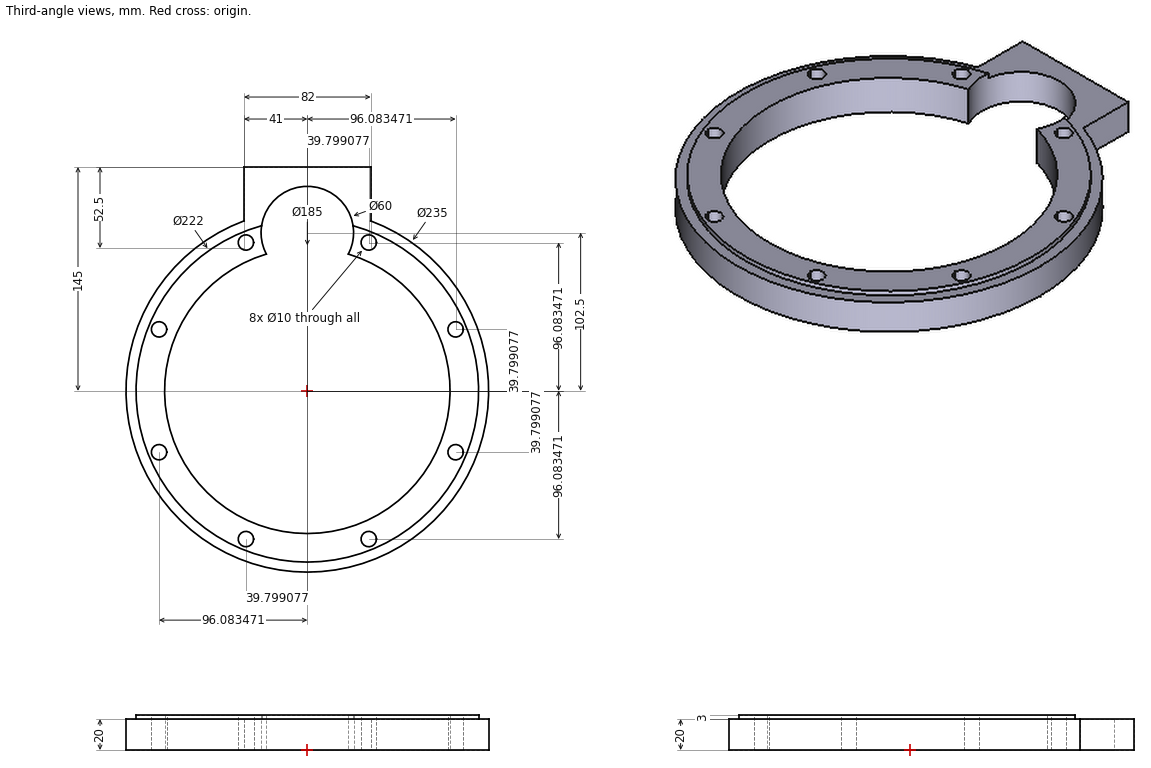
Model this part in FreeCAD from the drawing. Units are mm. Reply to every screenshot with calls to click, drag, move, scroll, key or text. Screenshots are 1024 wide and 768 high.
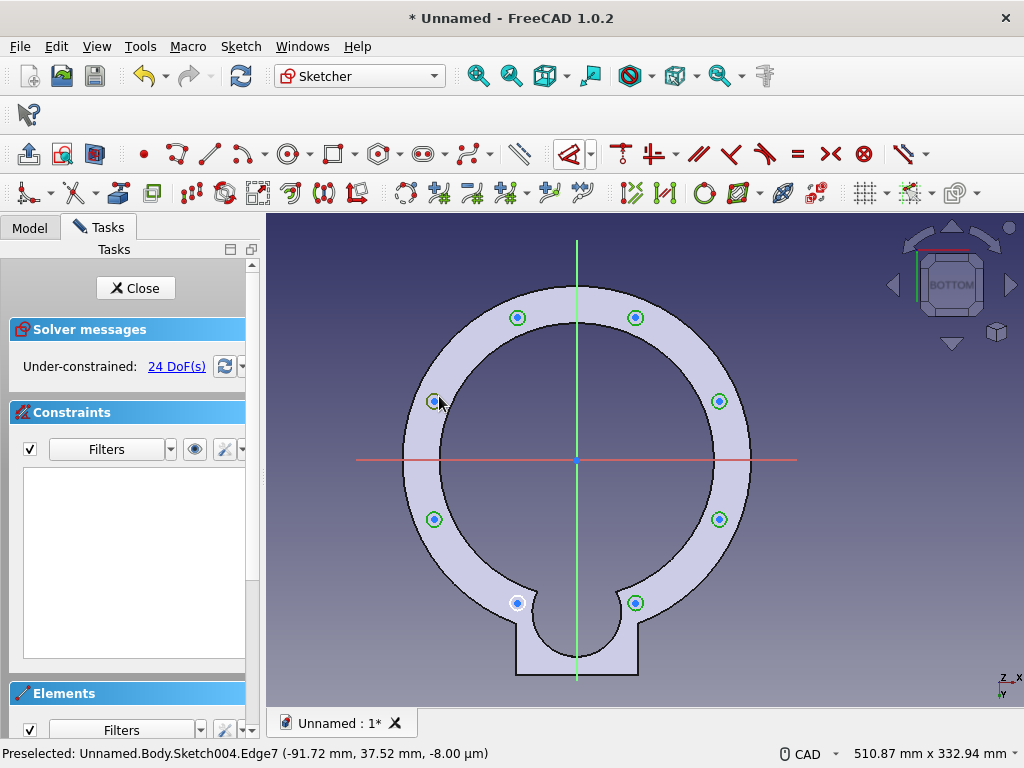
scroll(523, 598, up, 4)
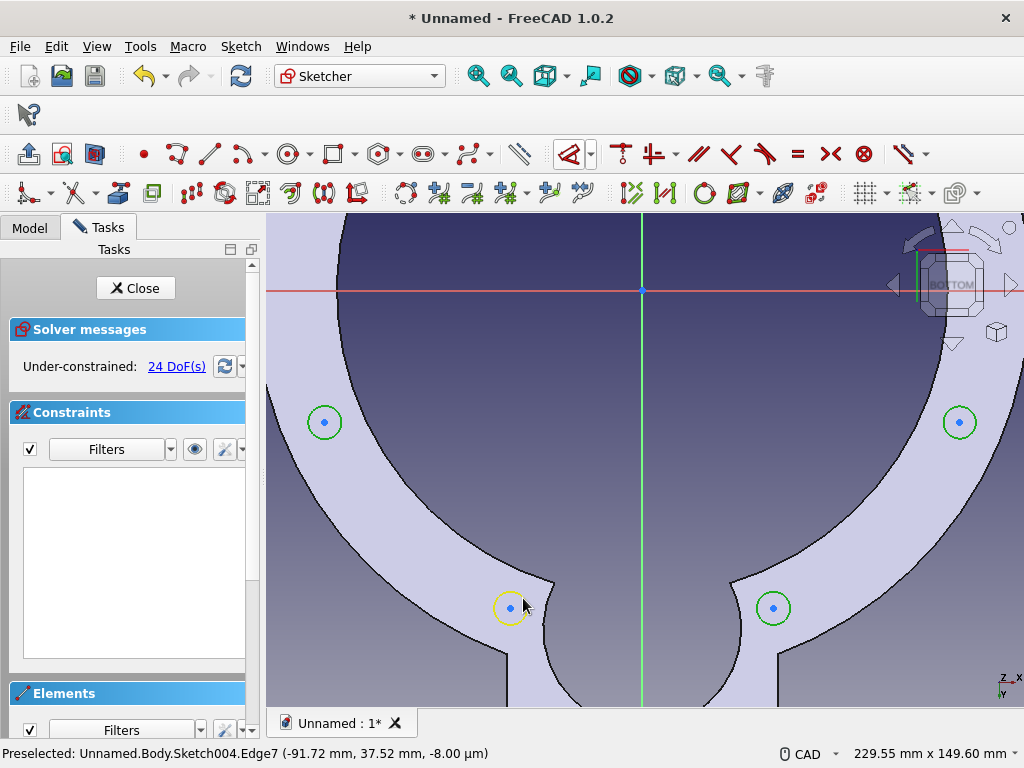
click(522, 597)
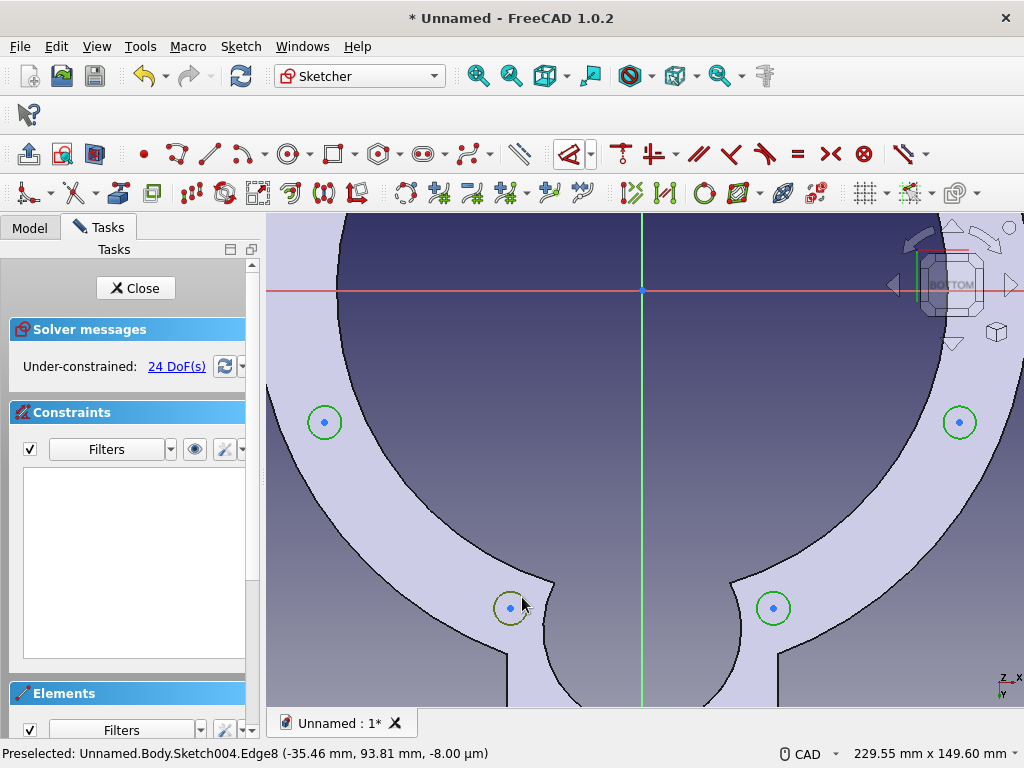
click(798, 154)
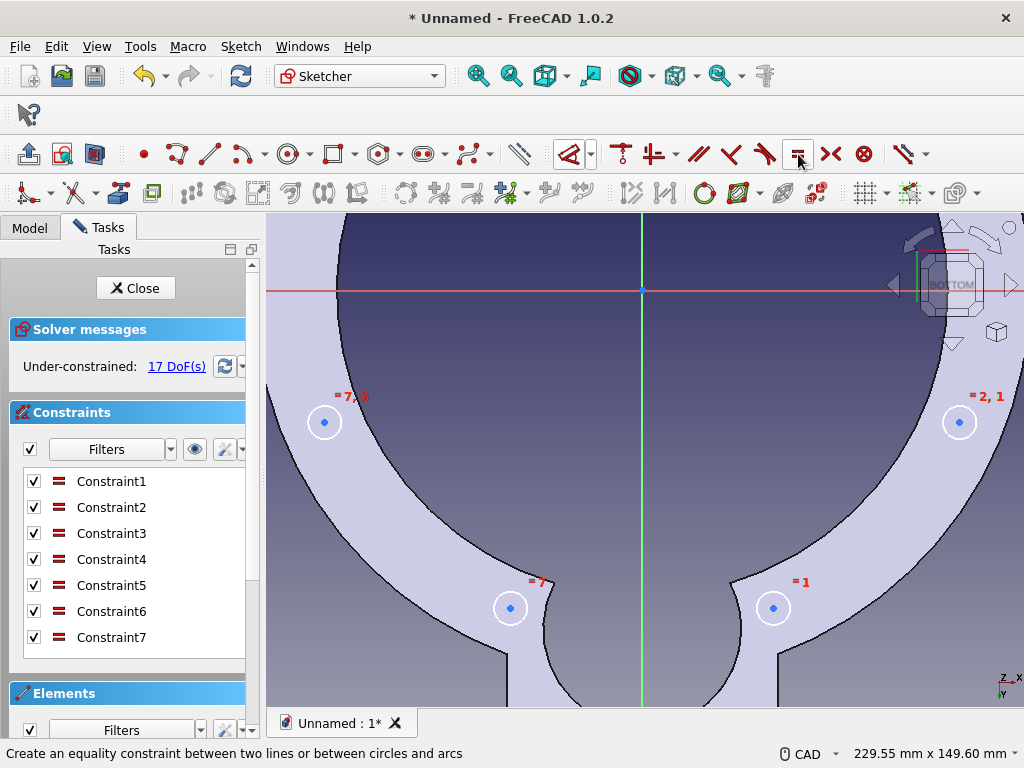
scroll(523, 598, down, 4)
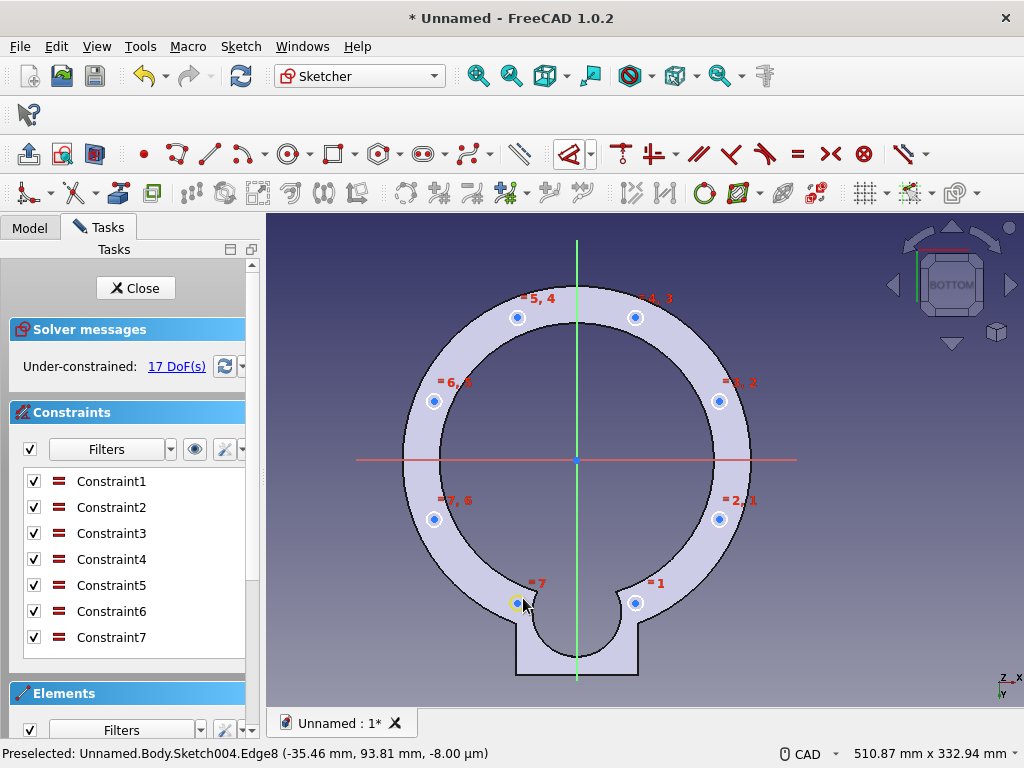
click(719, 520)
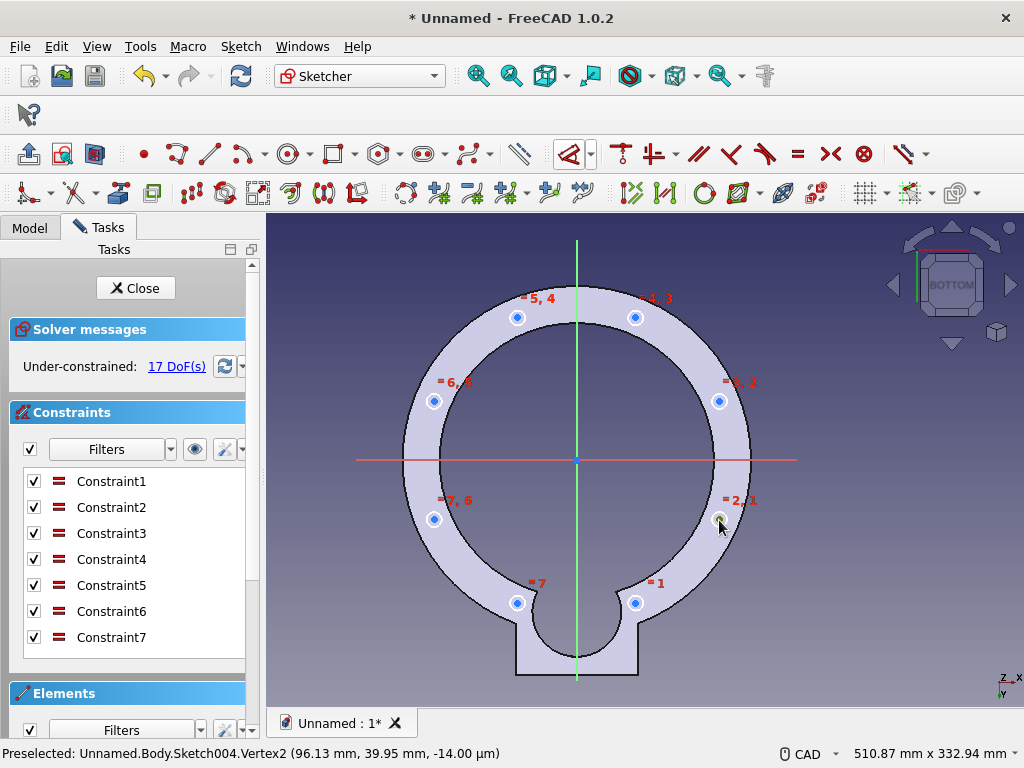
click(719, 401)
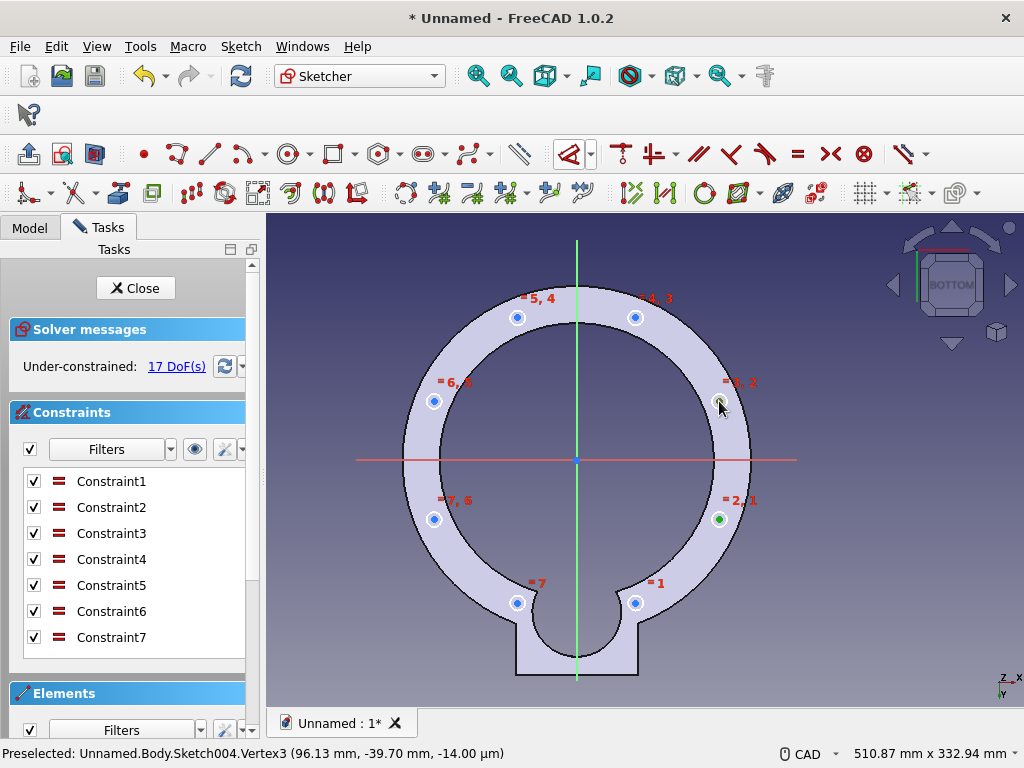
click(676, 154)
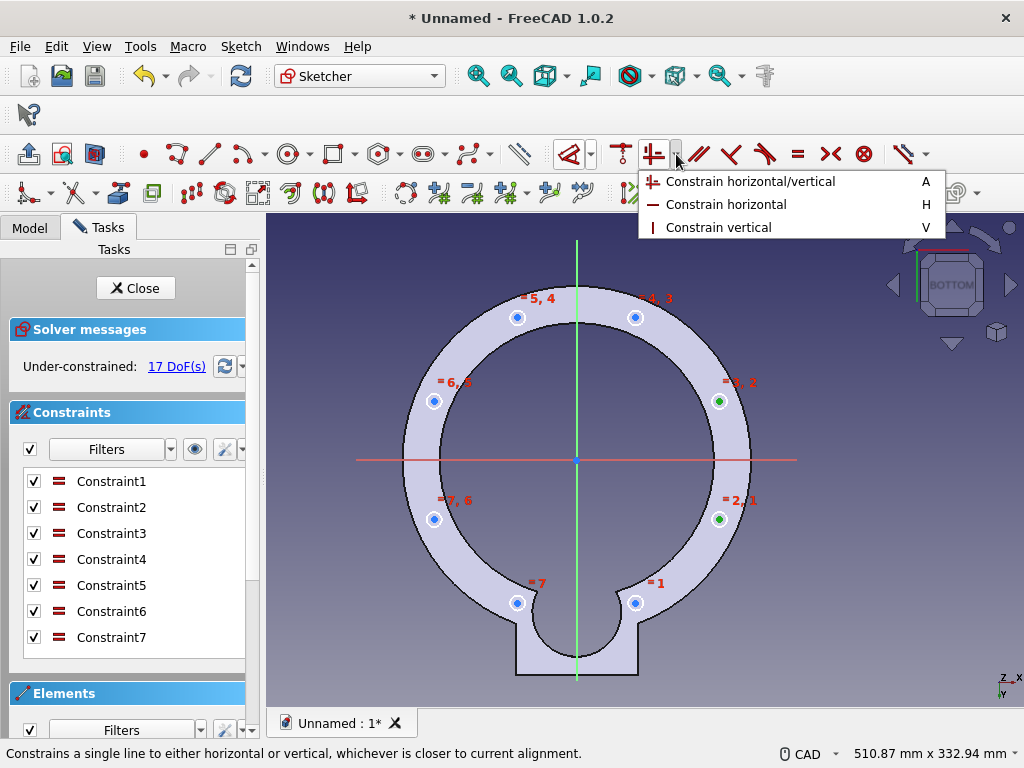
click(792, 228)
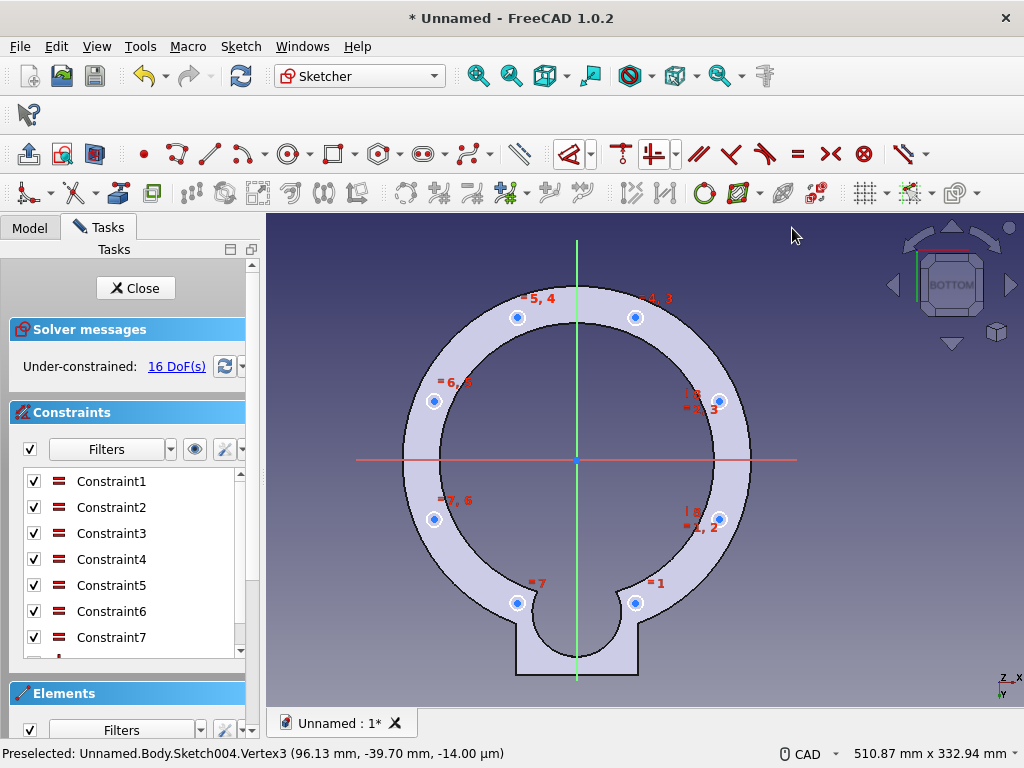
click(636, 603)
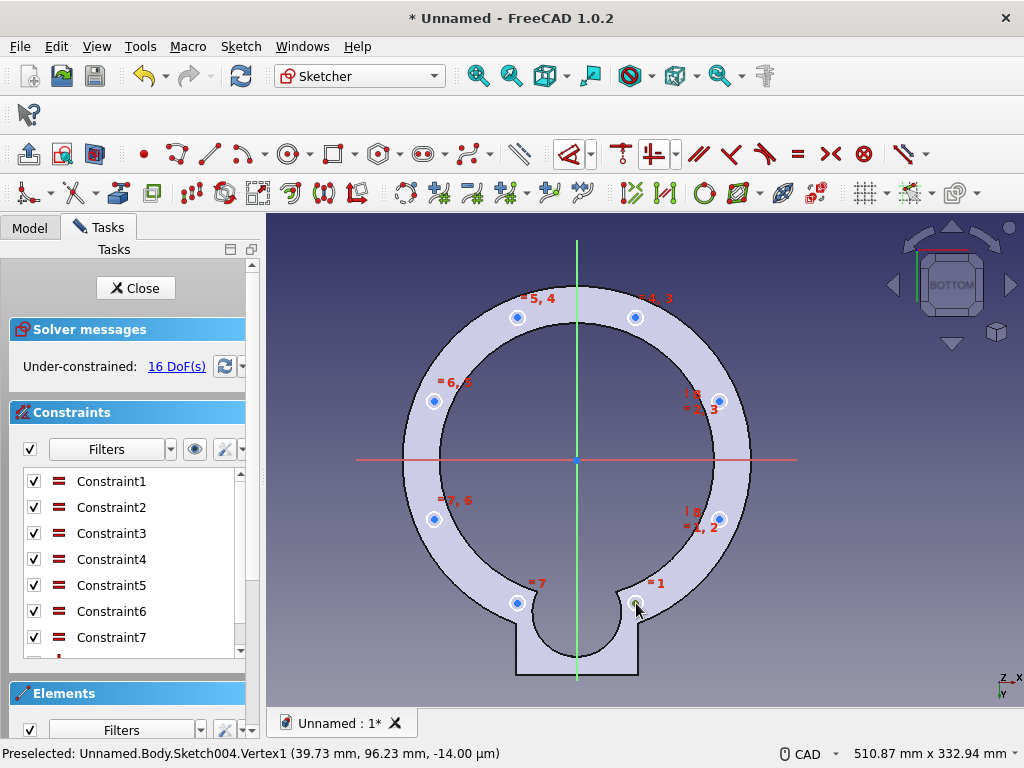
click(636, 318)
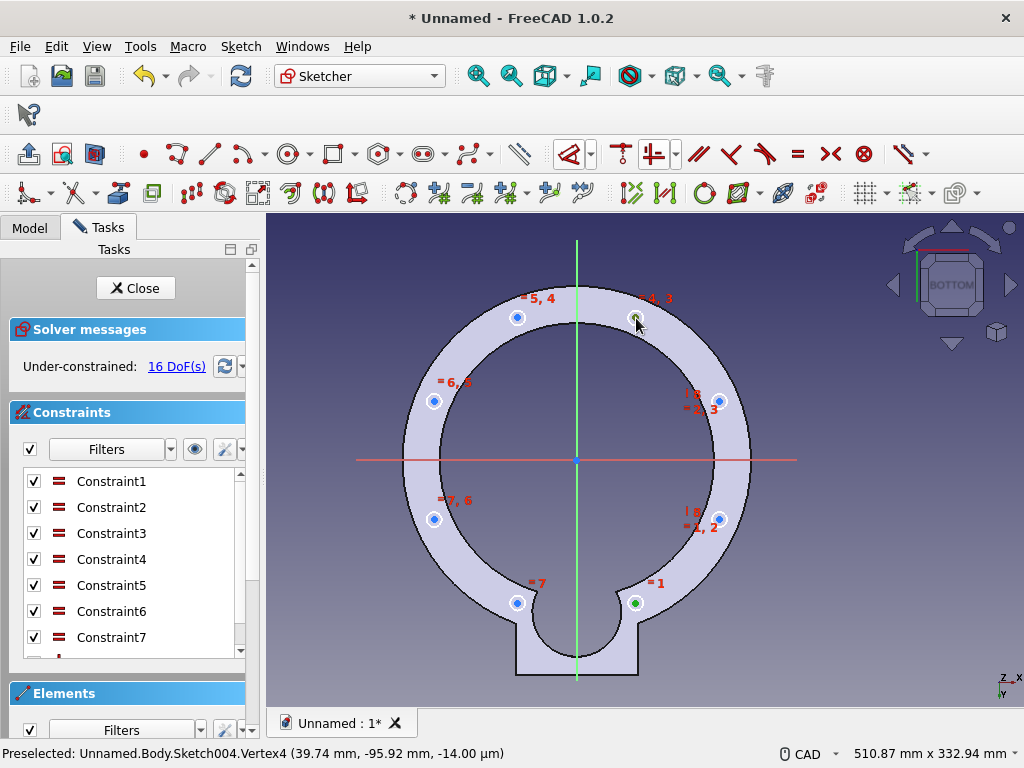
click(676, 154)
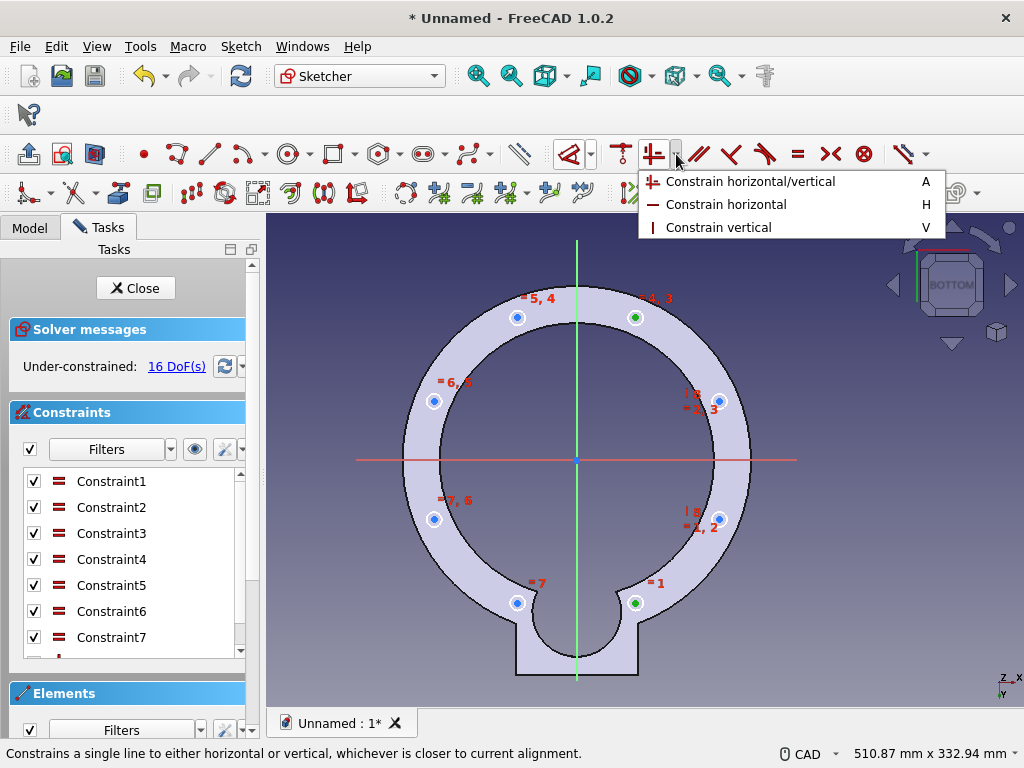
click(792, 228)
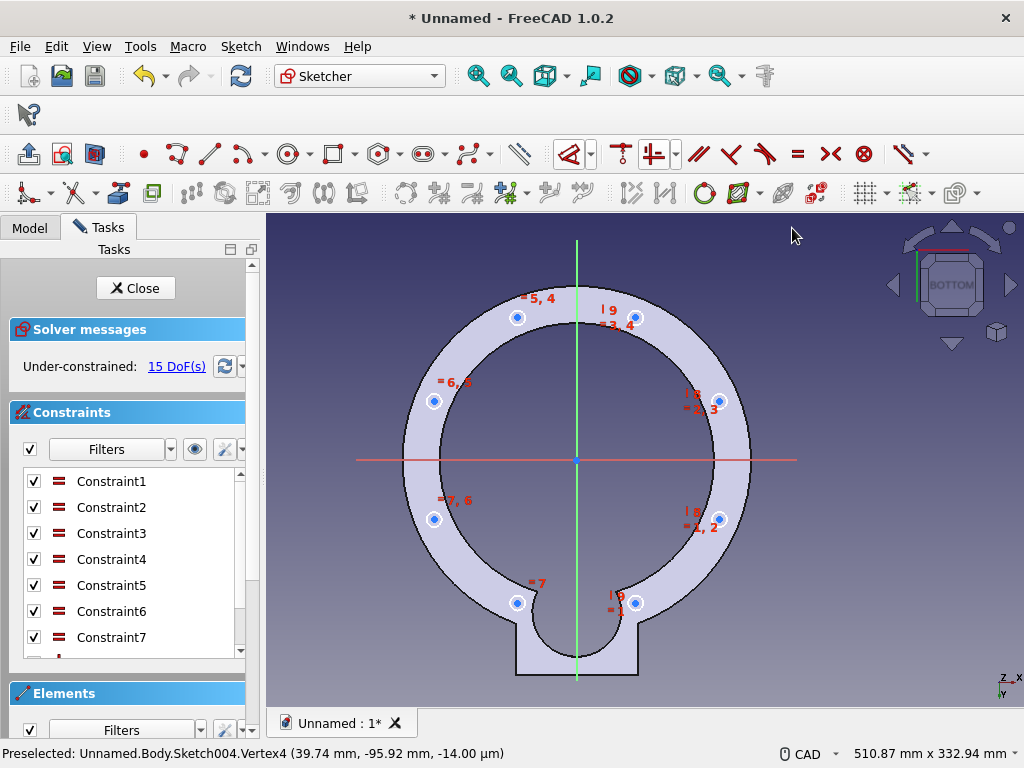
click(636, 318)